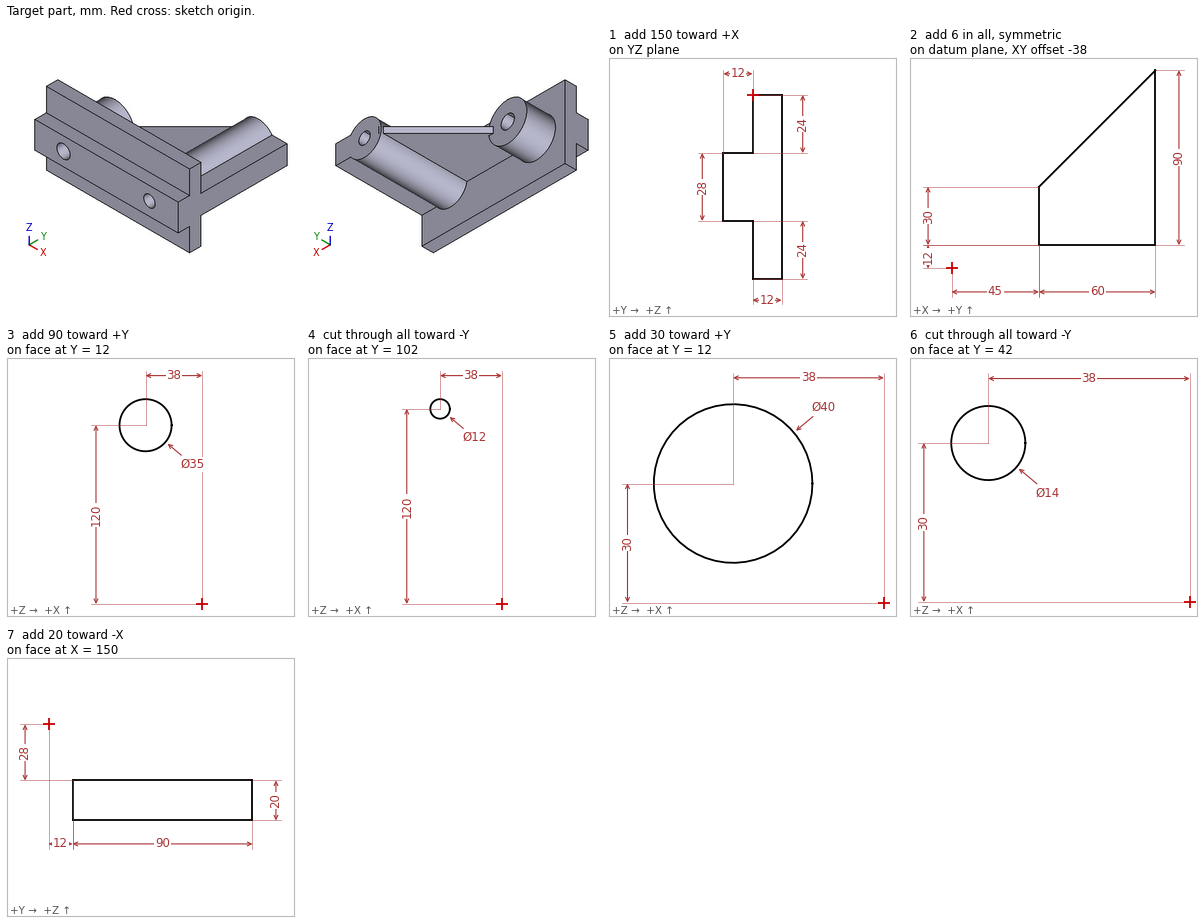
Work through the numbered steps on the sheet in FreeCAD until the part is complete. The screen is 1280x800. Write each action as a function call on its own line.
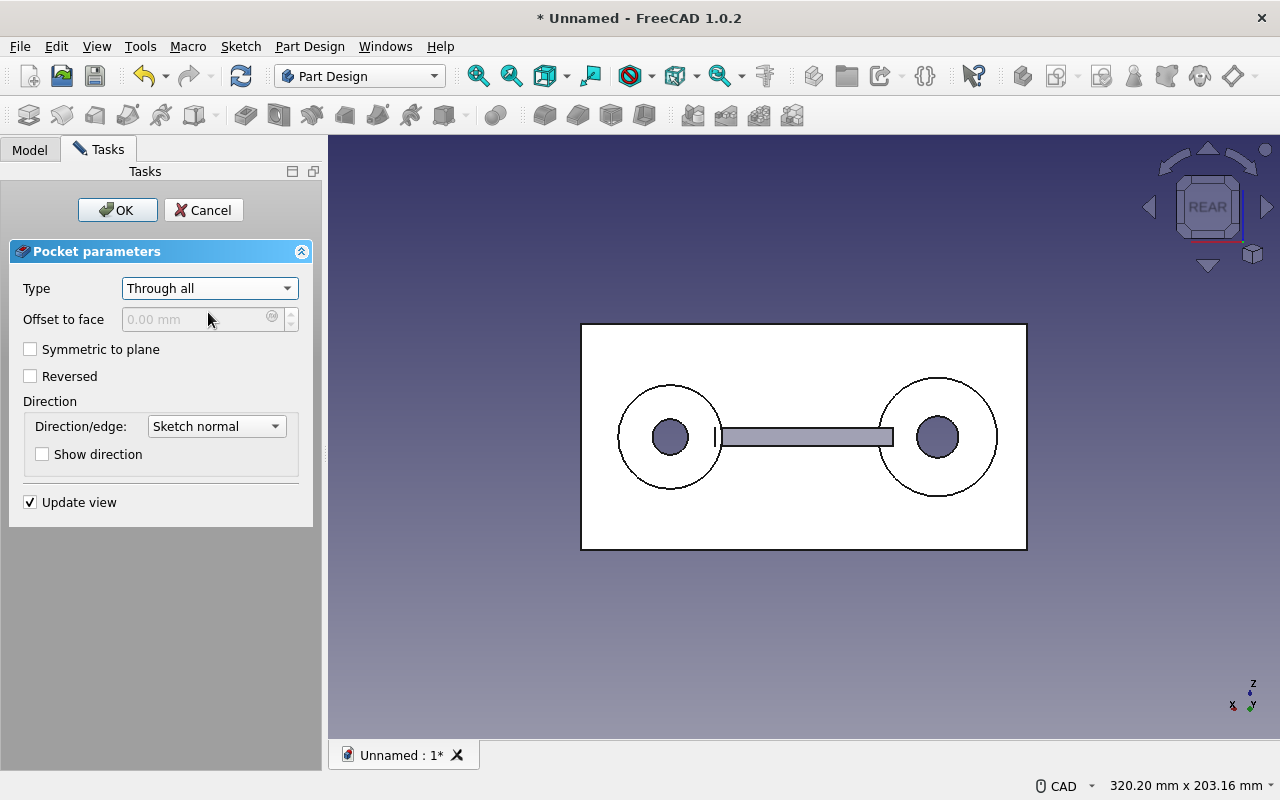
click(118, 210)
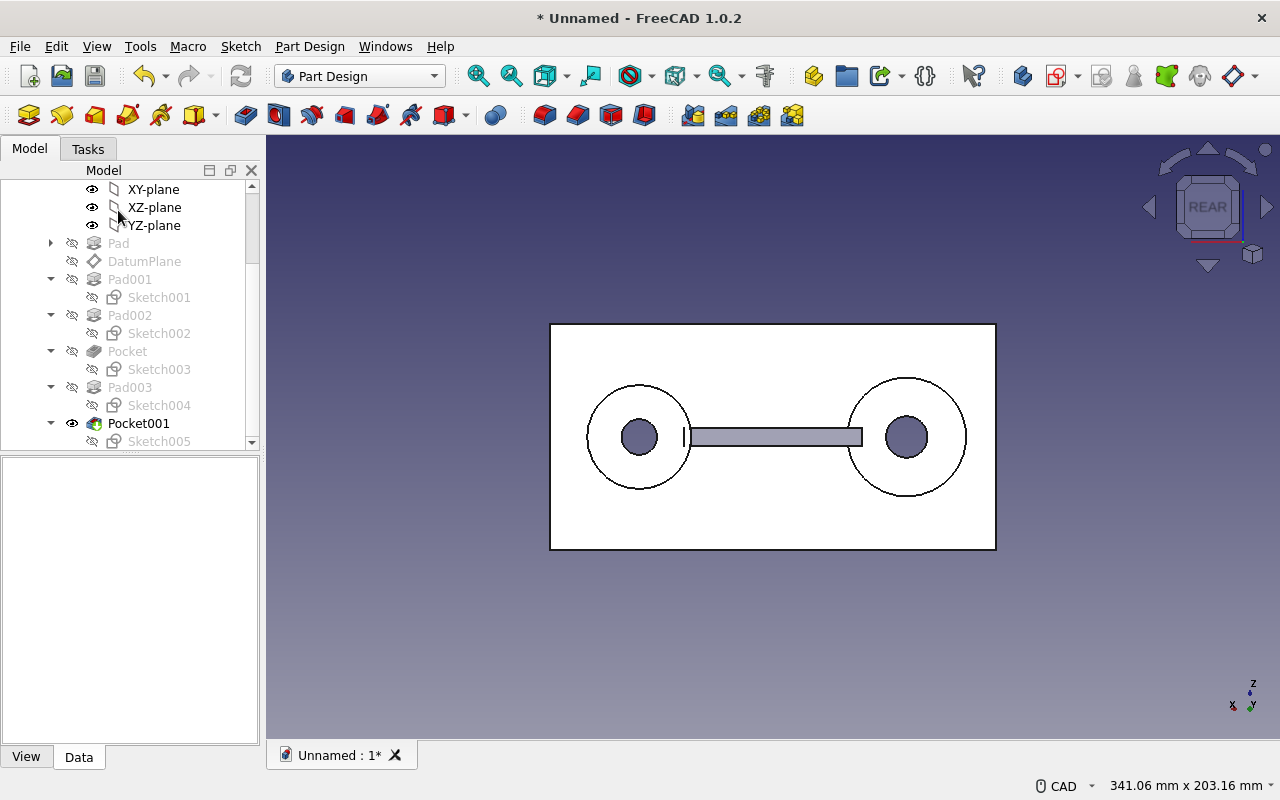
click(479, 76)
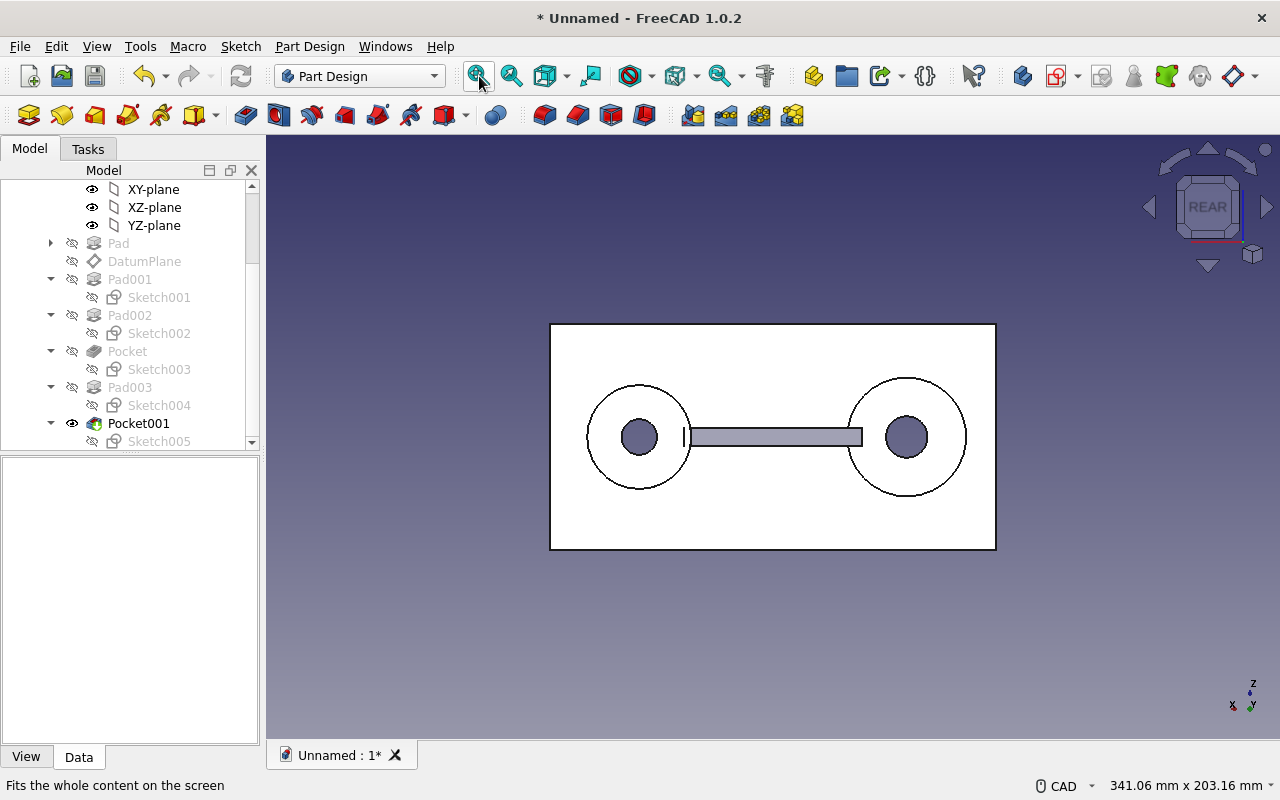
key(0)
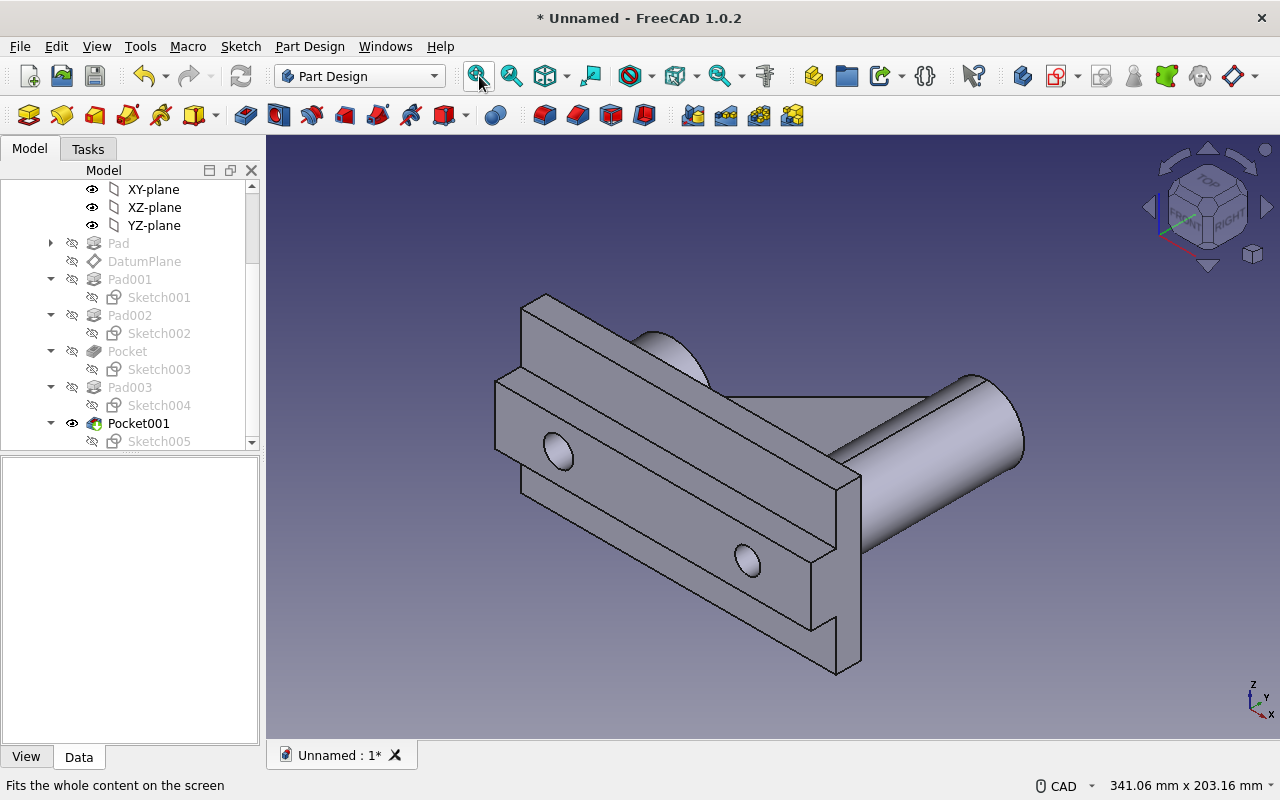
click(836, 582)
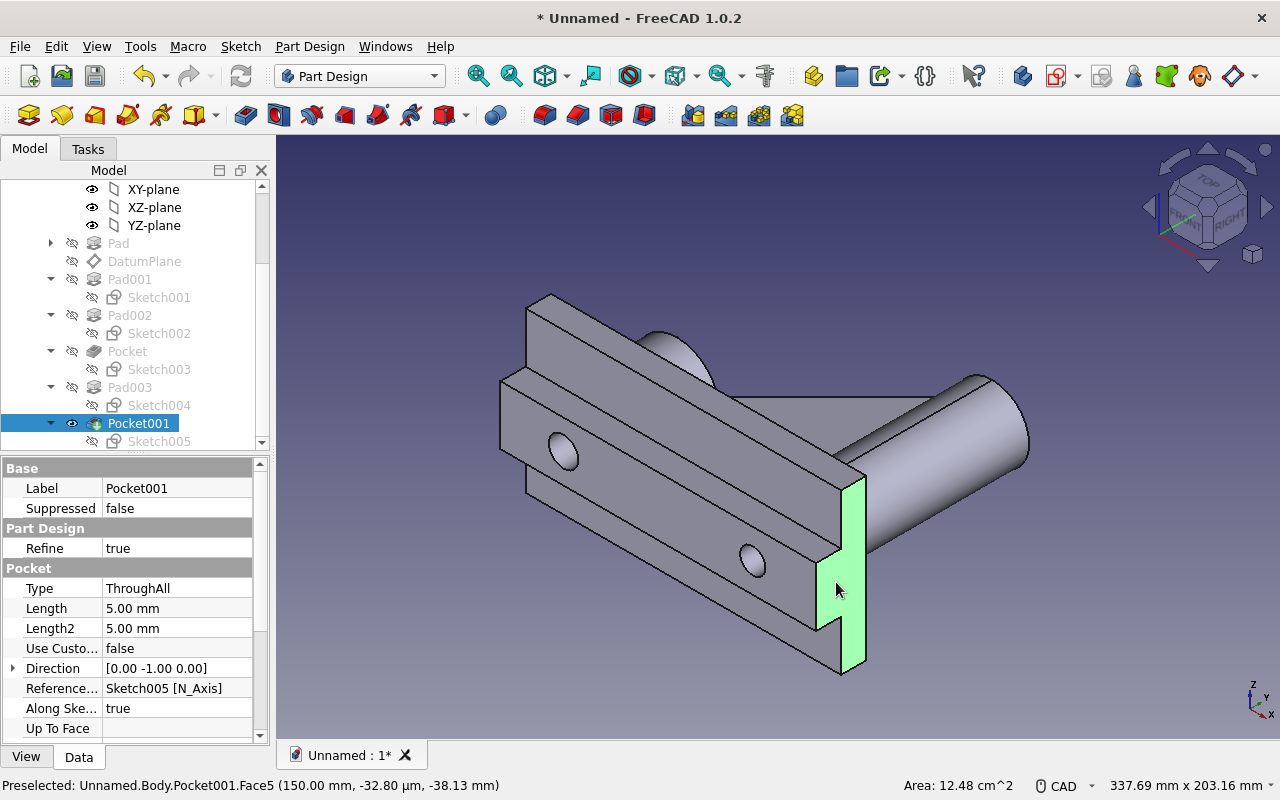
click(1056, 76)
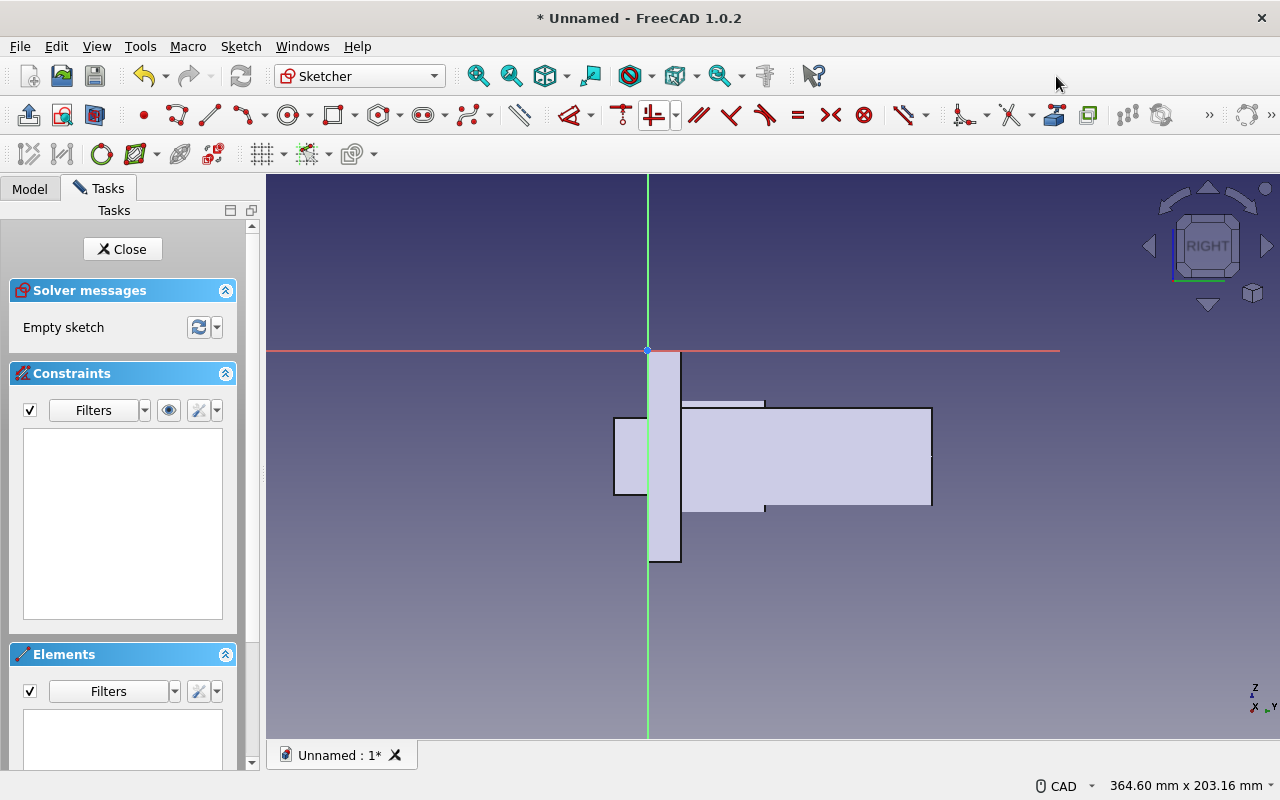
scroll(859, 386, up, 4)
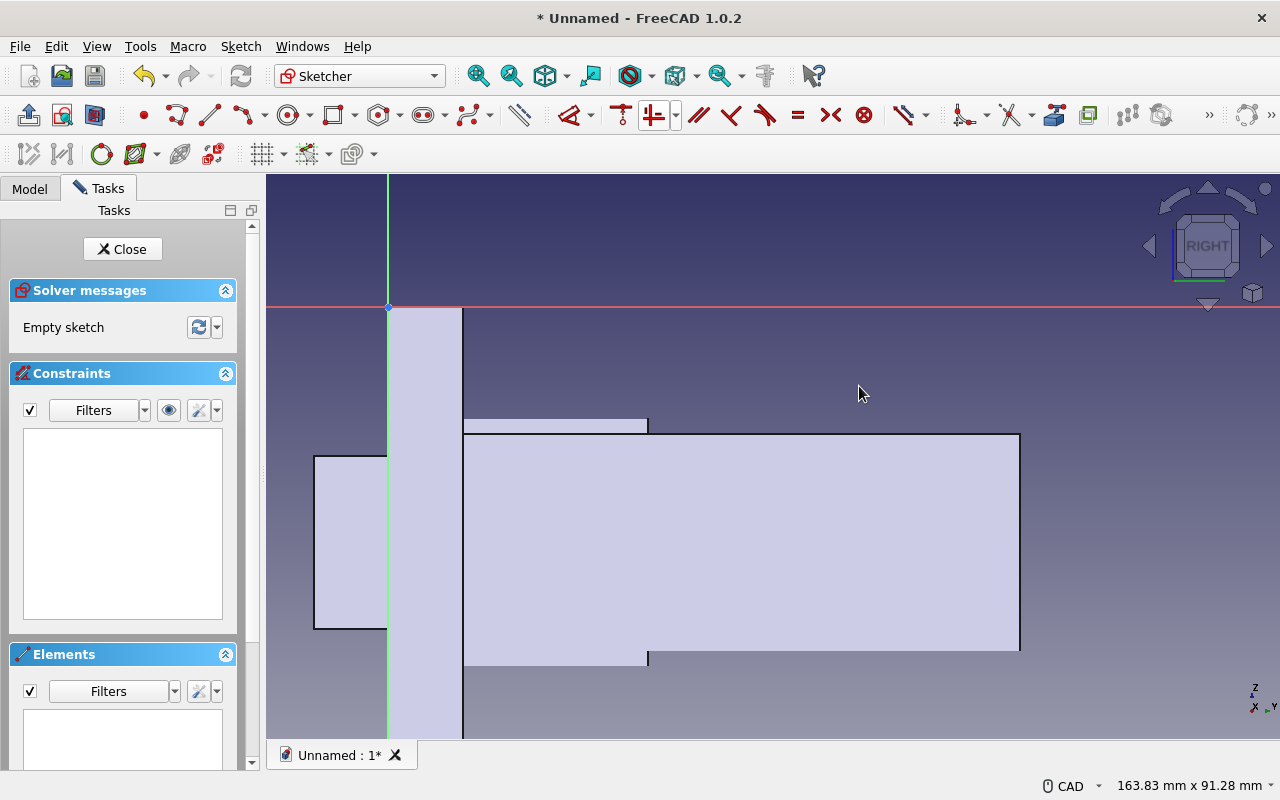
click(332, 116)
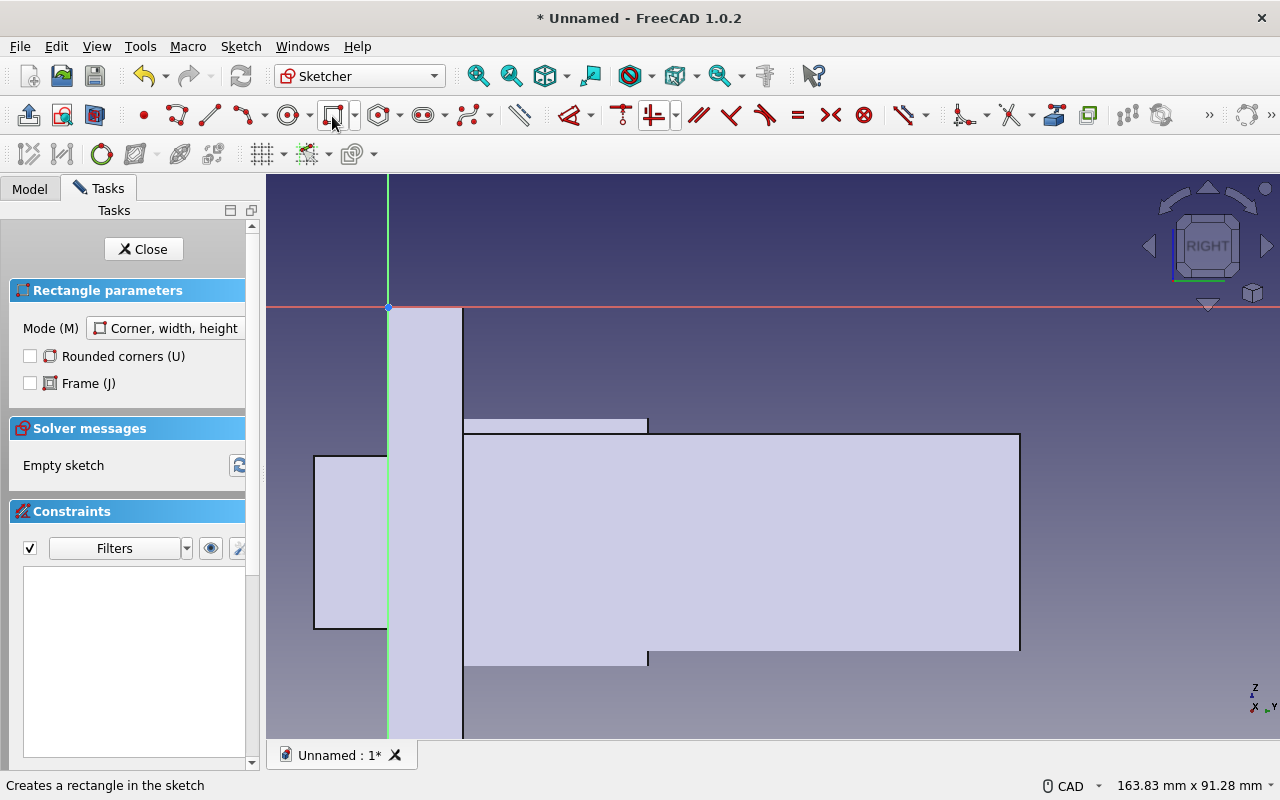
click(463, 481)
move(1020, 604)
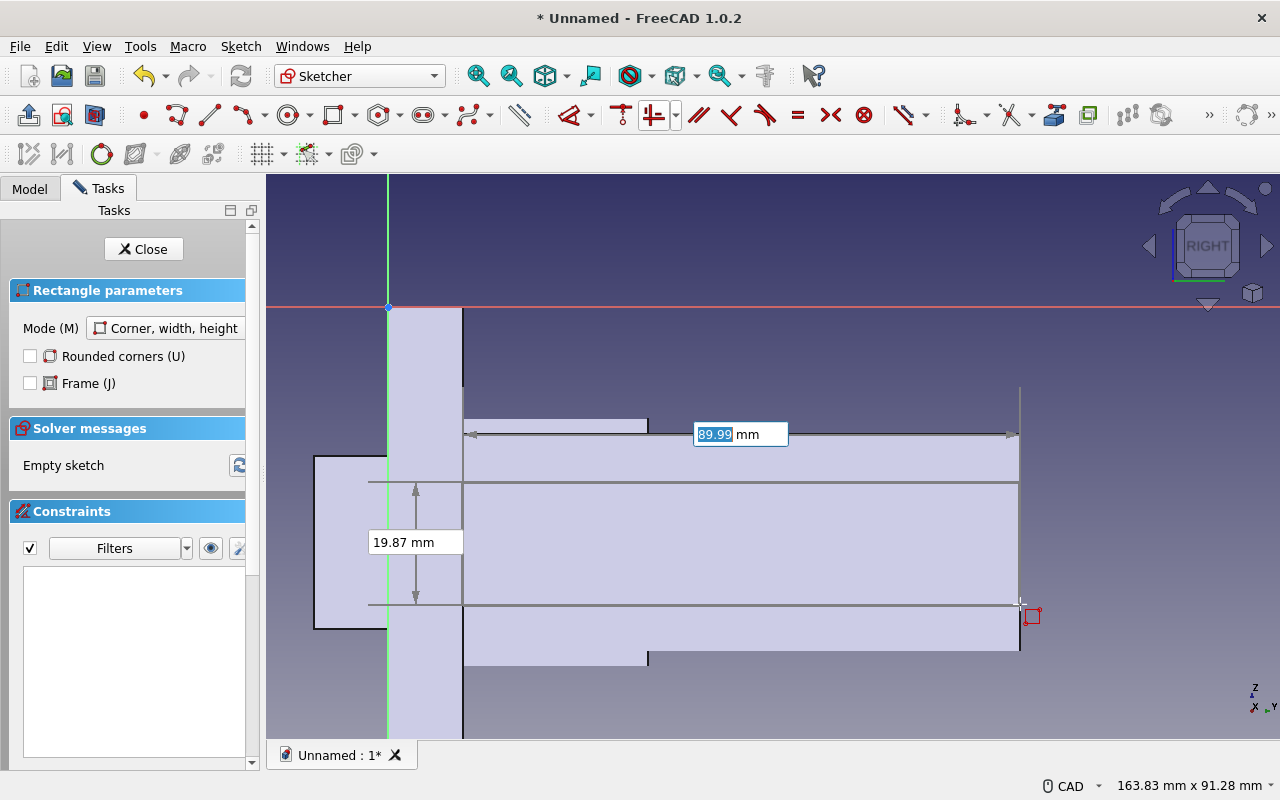
text(90)
key(Tab)
text(20)
key(Return)
key(Escape)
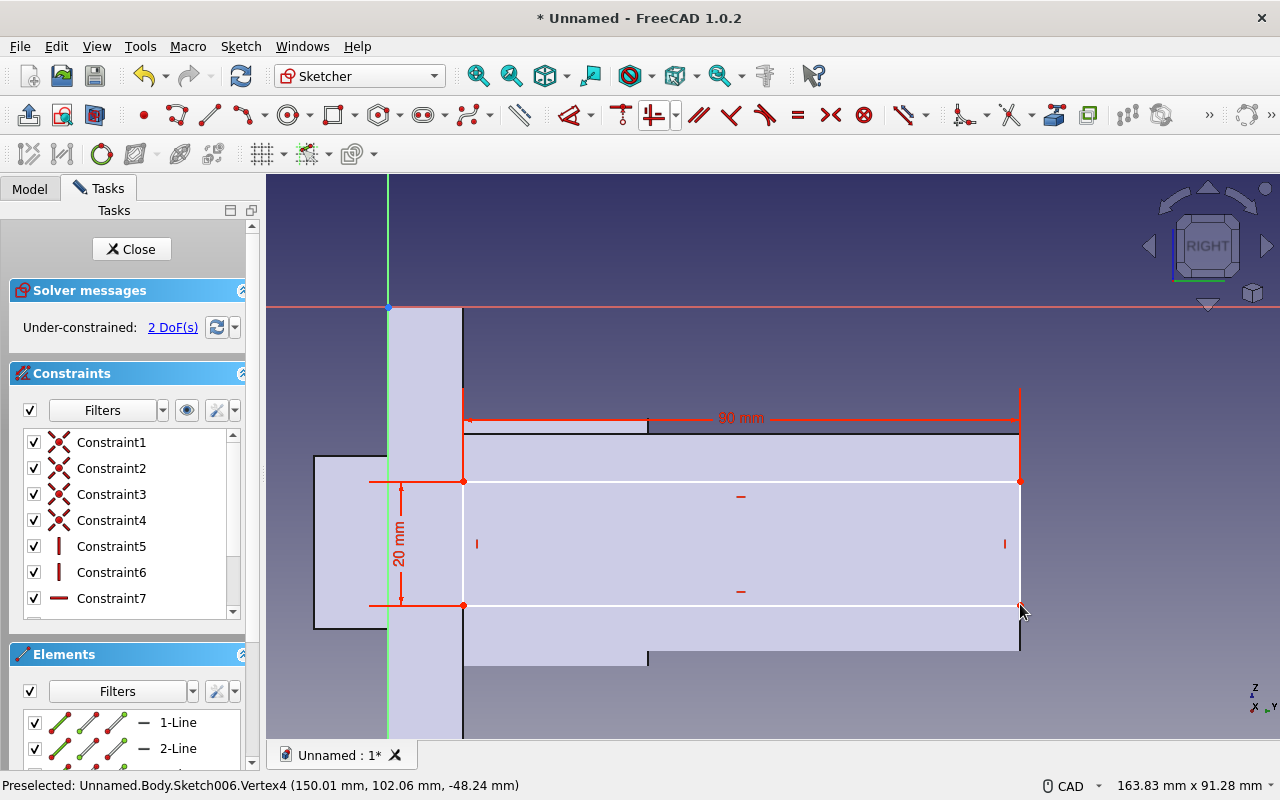
click(568, 116)